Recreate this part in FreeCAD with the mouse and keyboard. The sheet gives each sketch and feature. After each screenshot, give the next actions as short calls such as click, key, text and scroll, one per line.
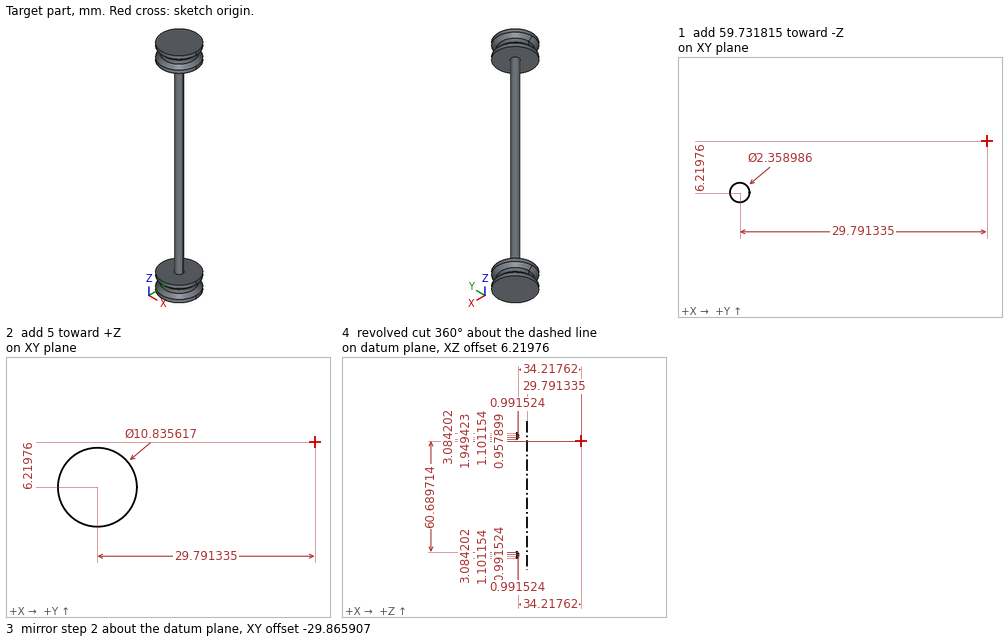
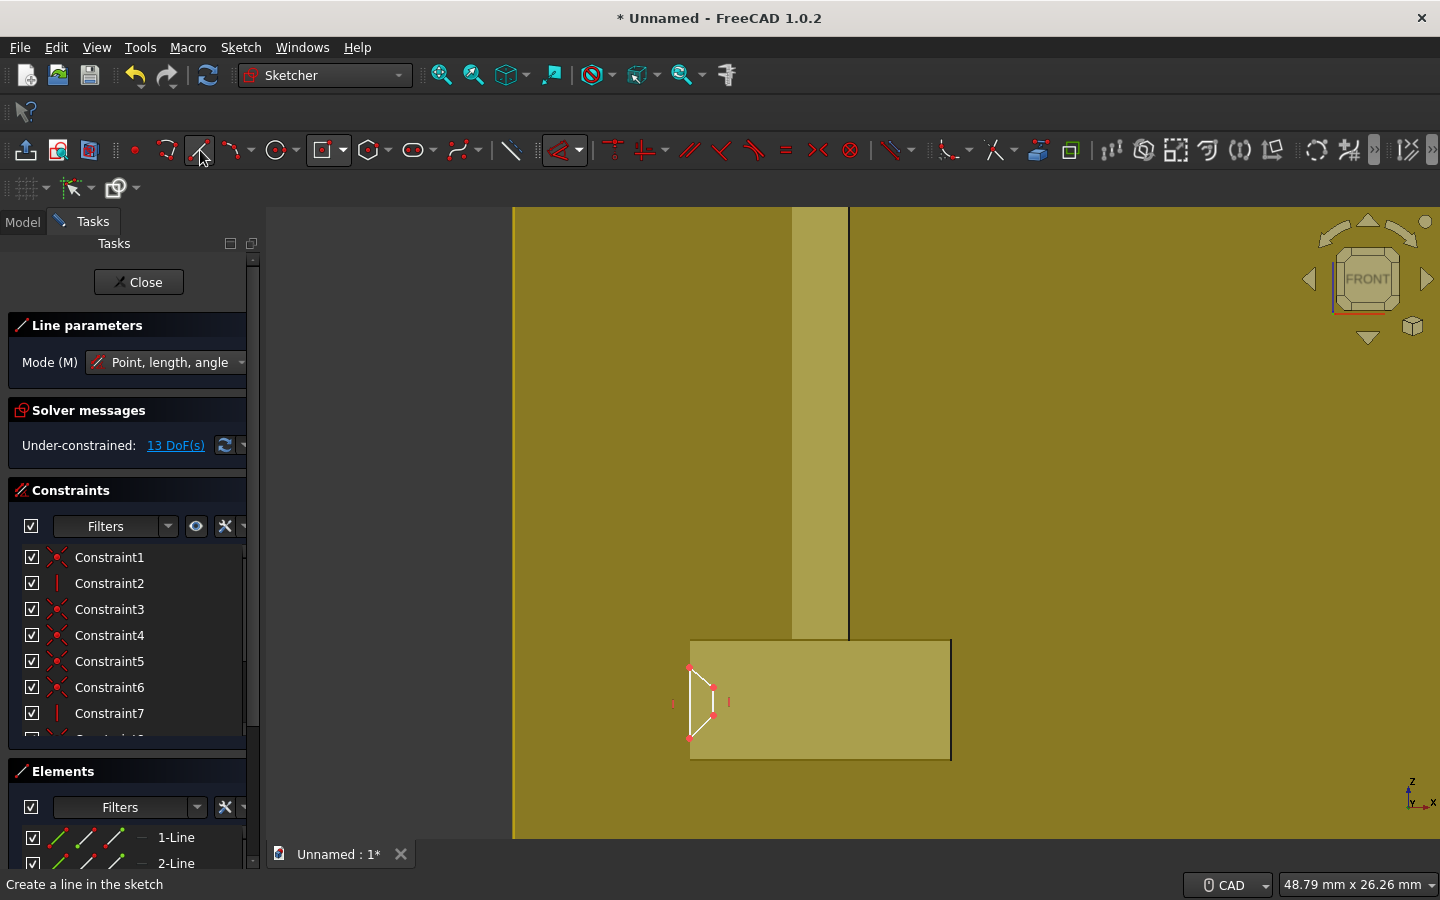
scroll(701, 675, down, 8)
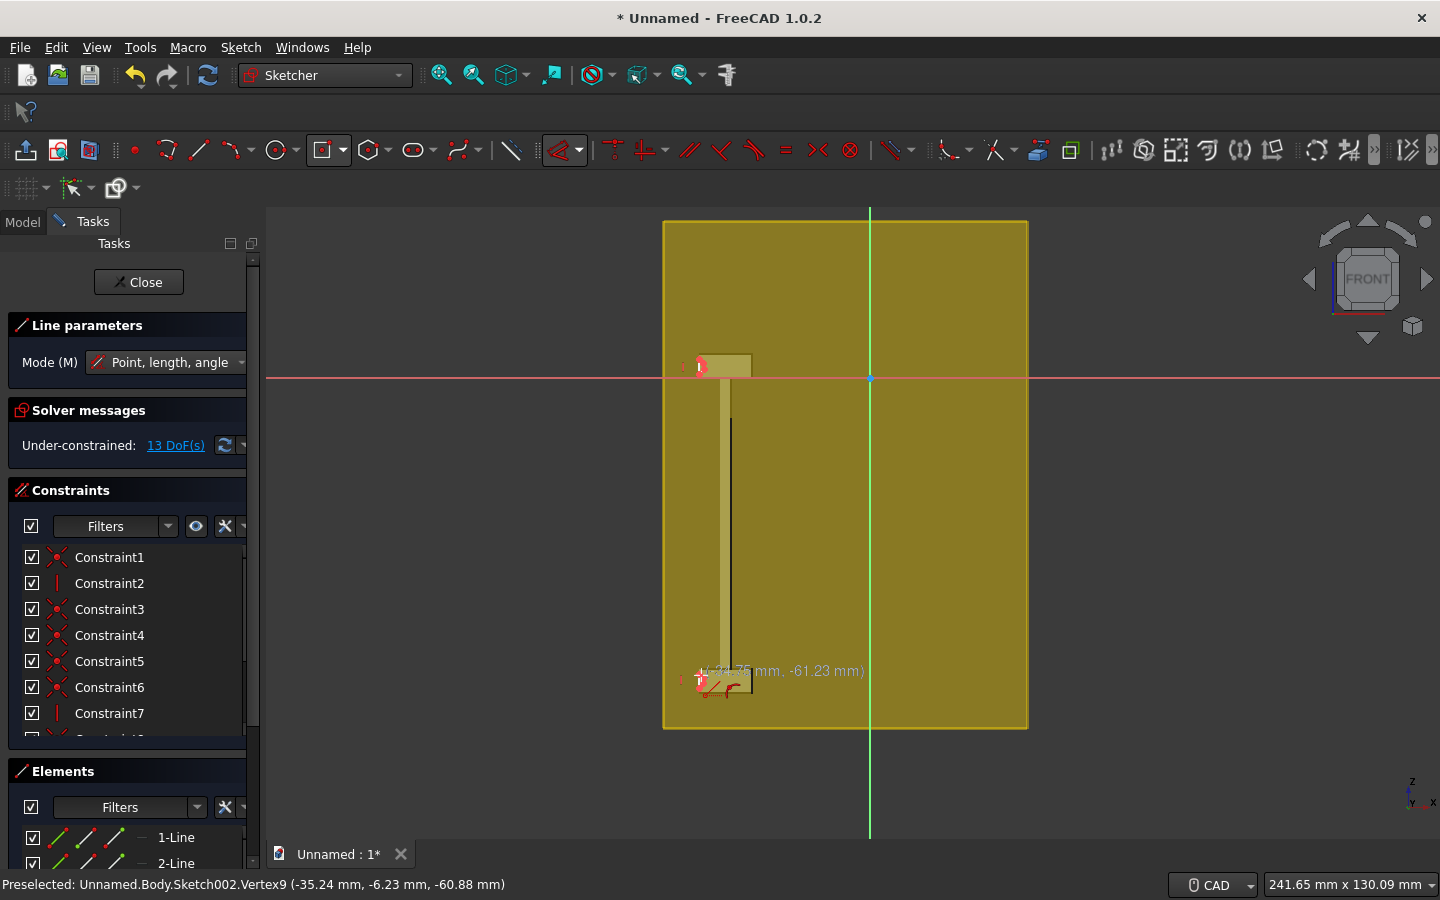
click(725, 326)
click(725, 721)
key(Escape)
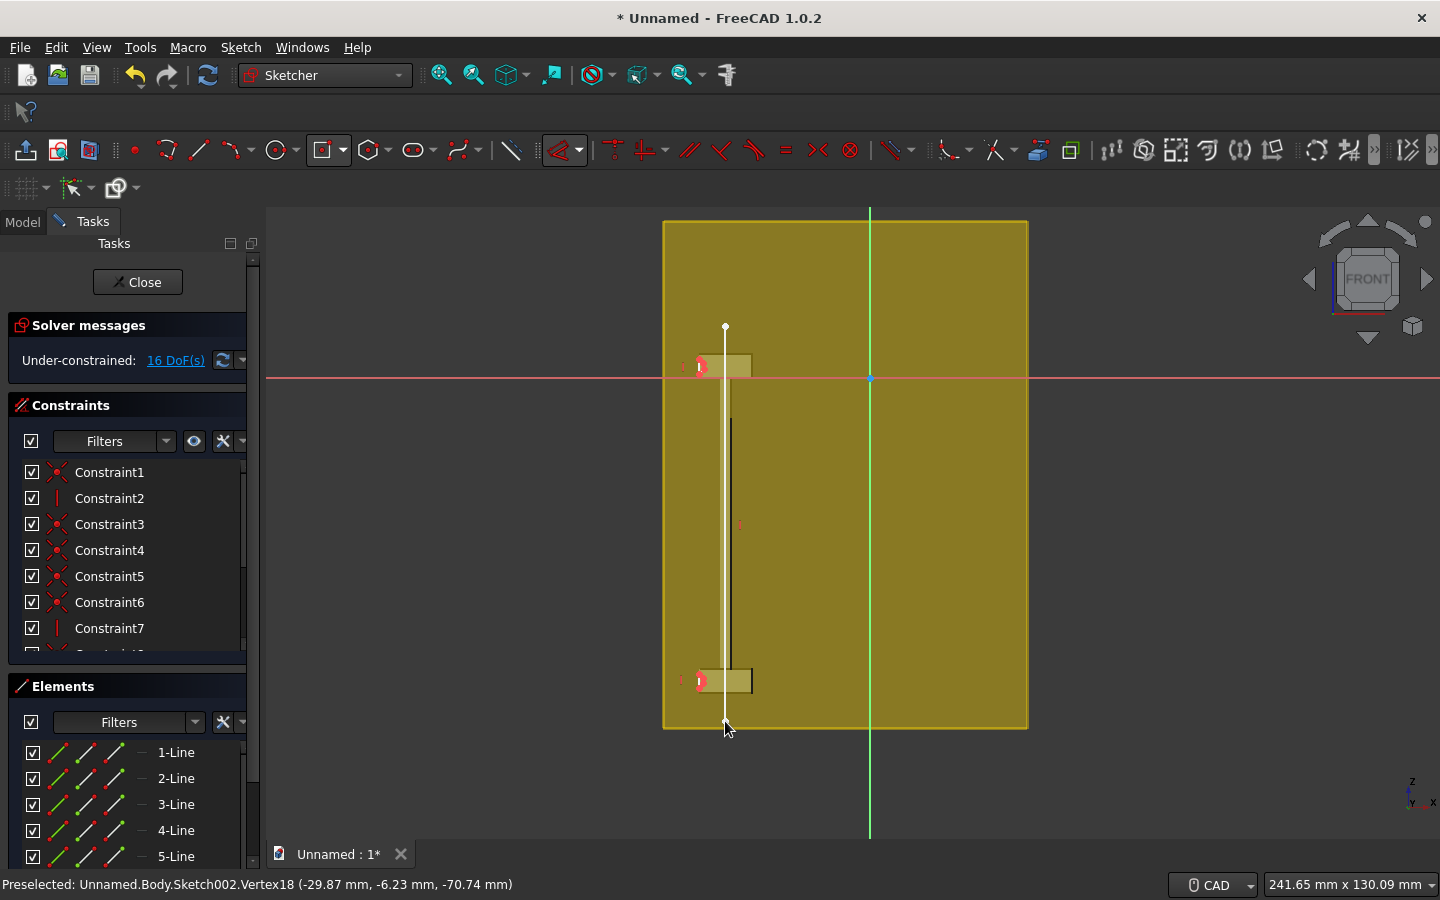
click(725, 445)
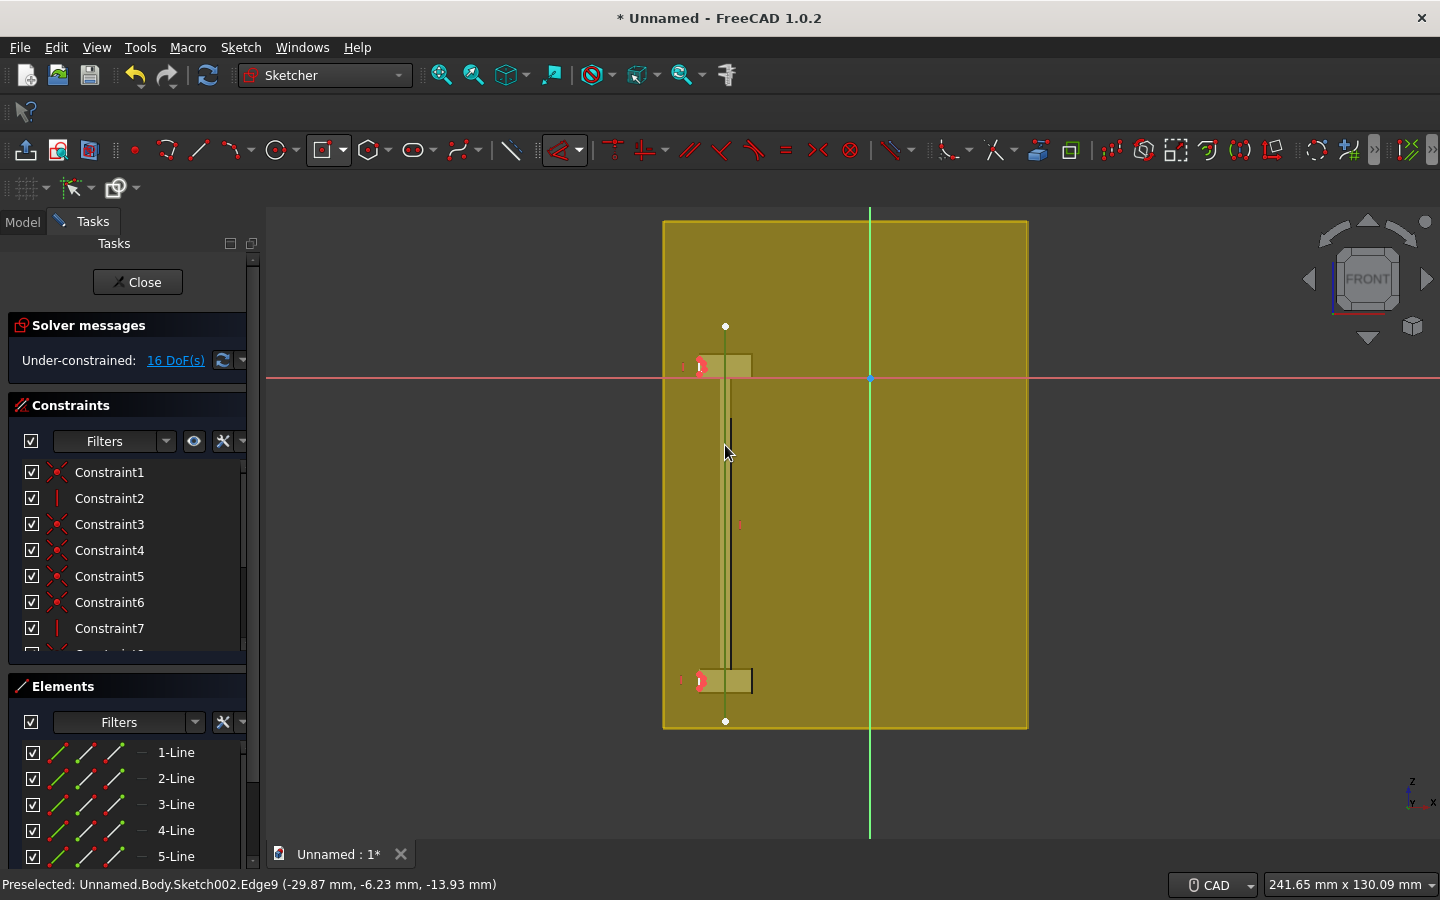
click(512, 150)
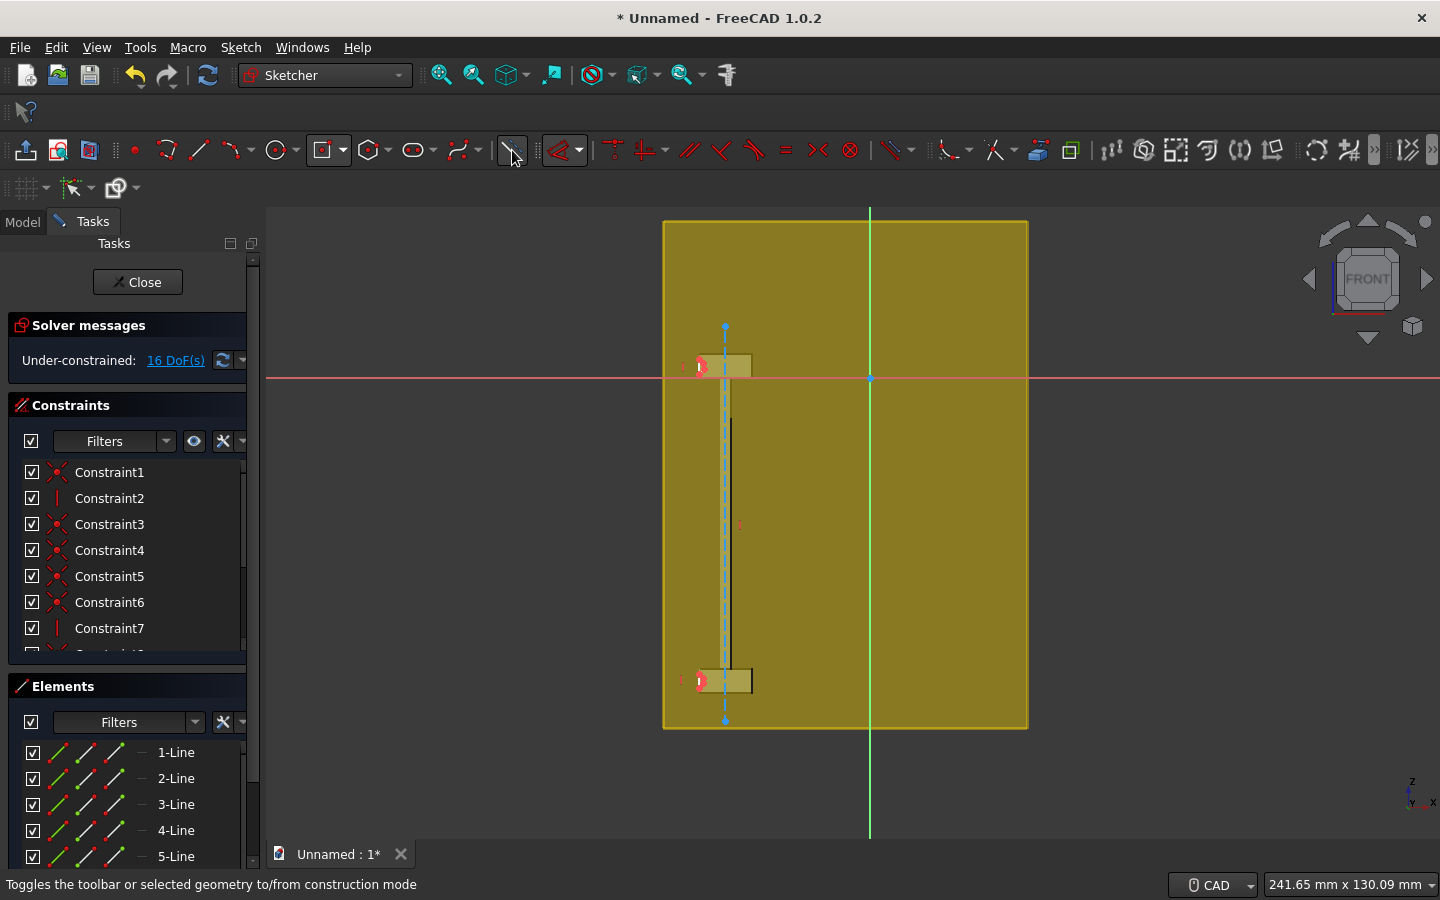
scroll(704, 367, up, 9)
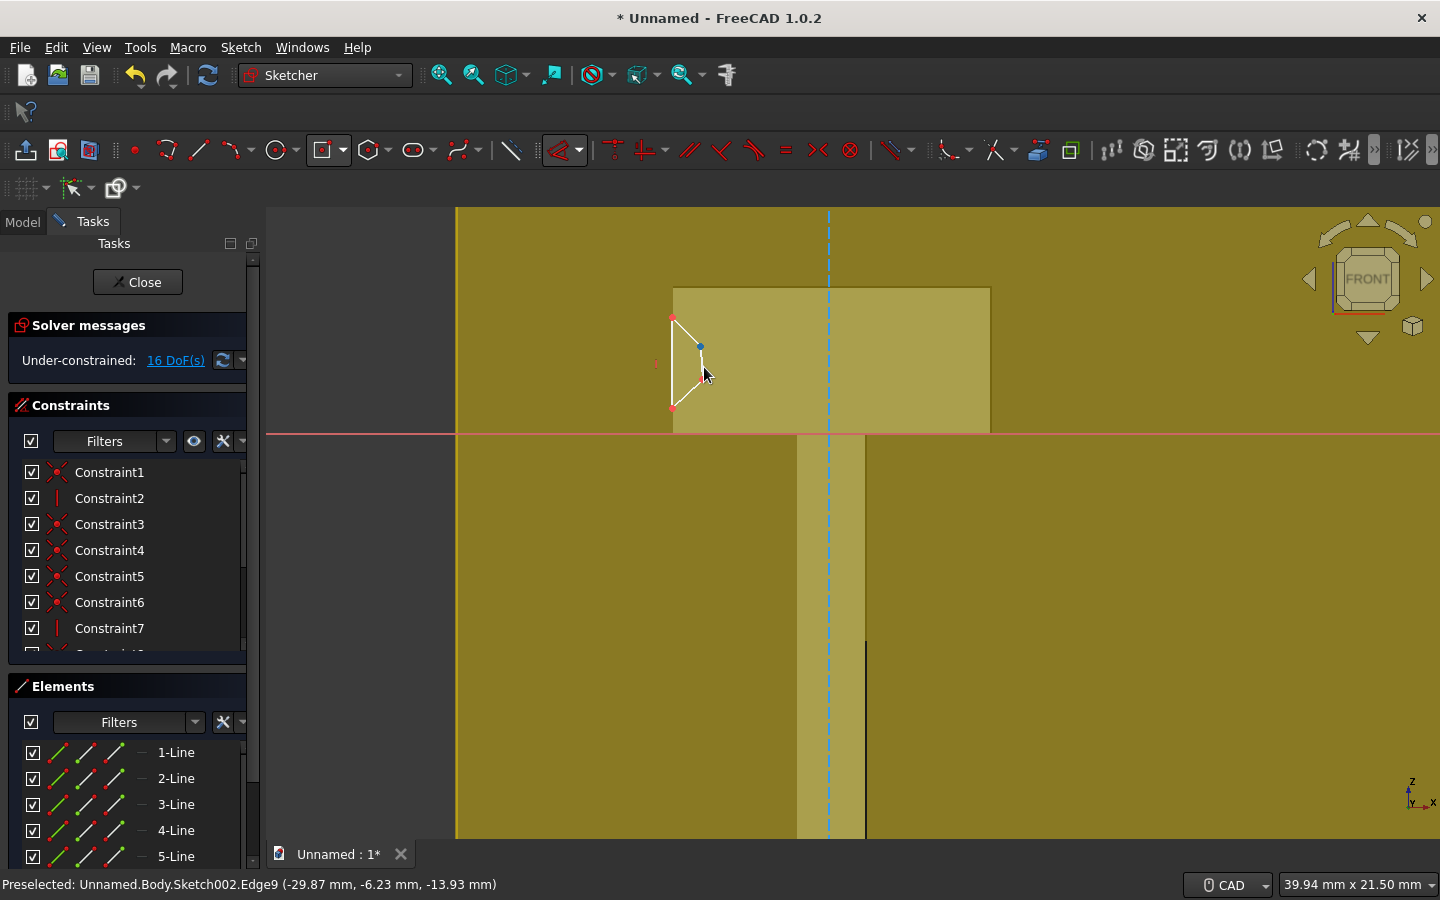
click(702, 363)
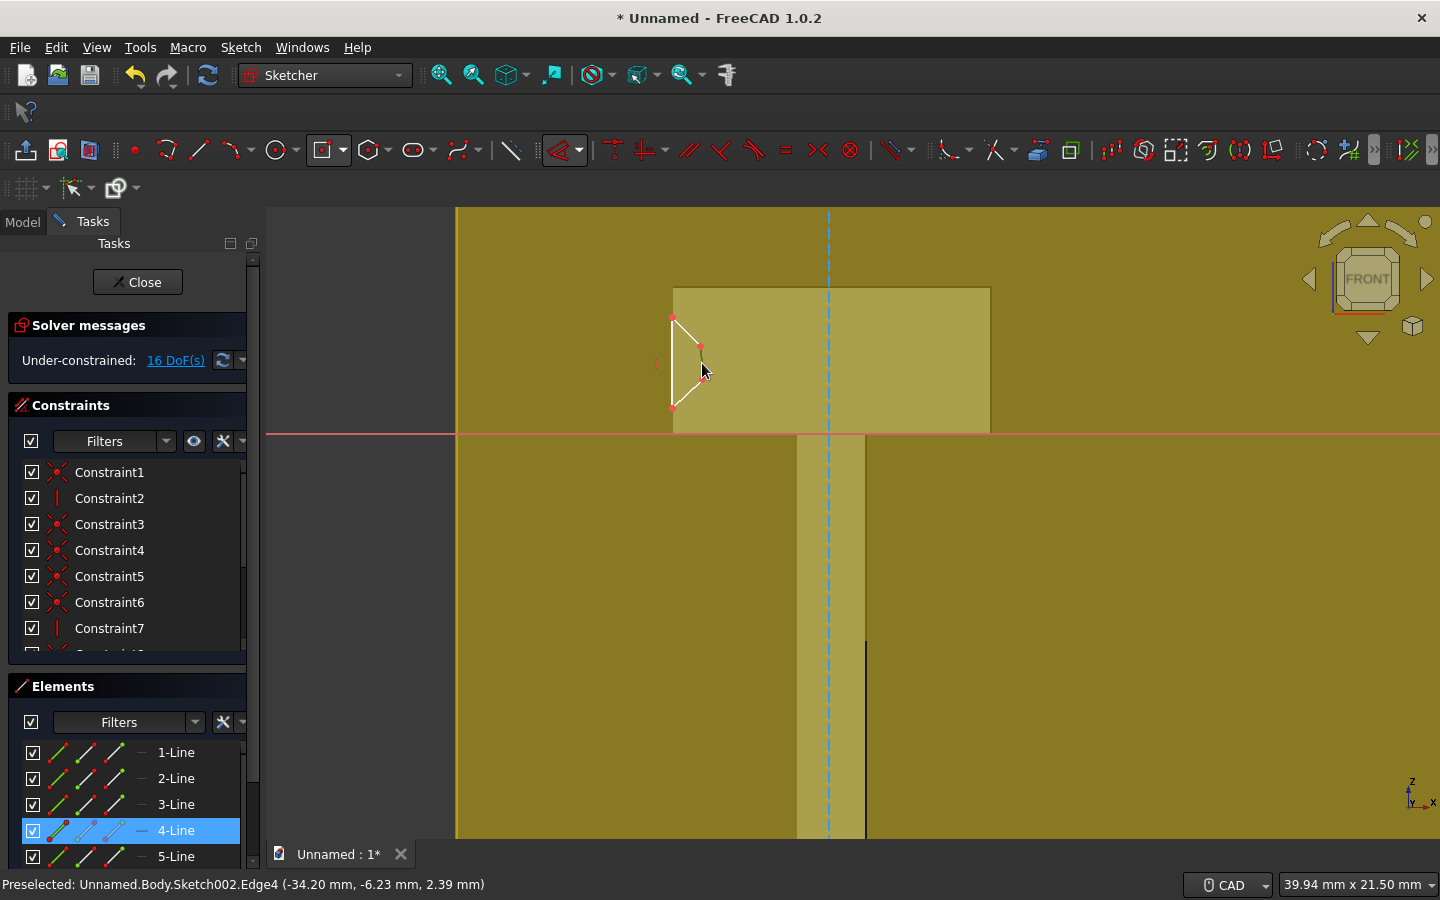
click(668, 150)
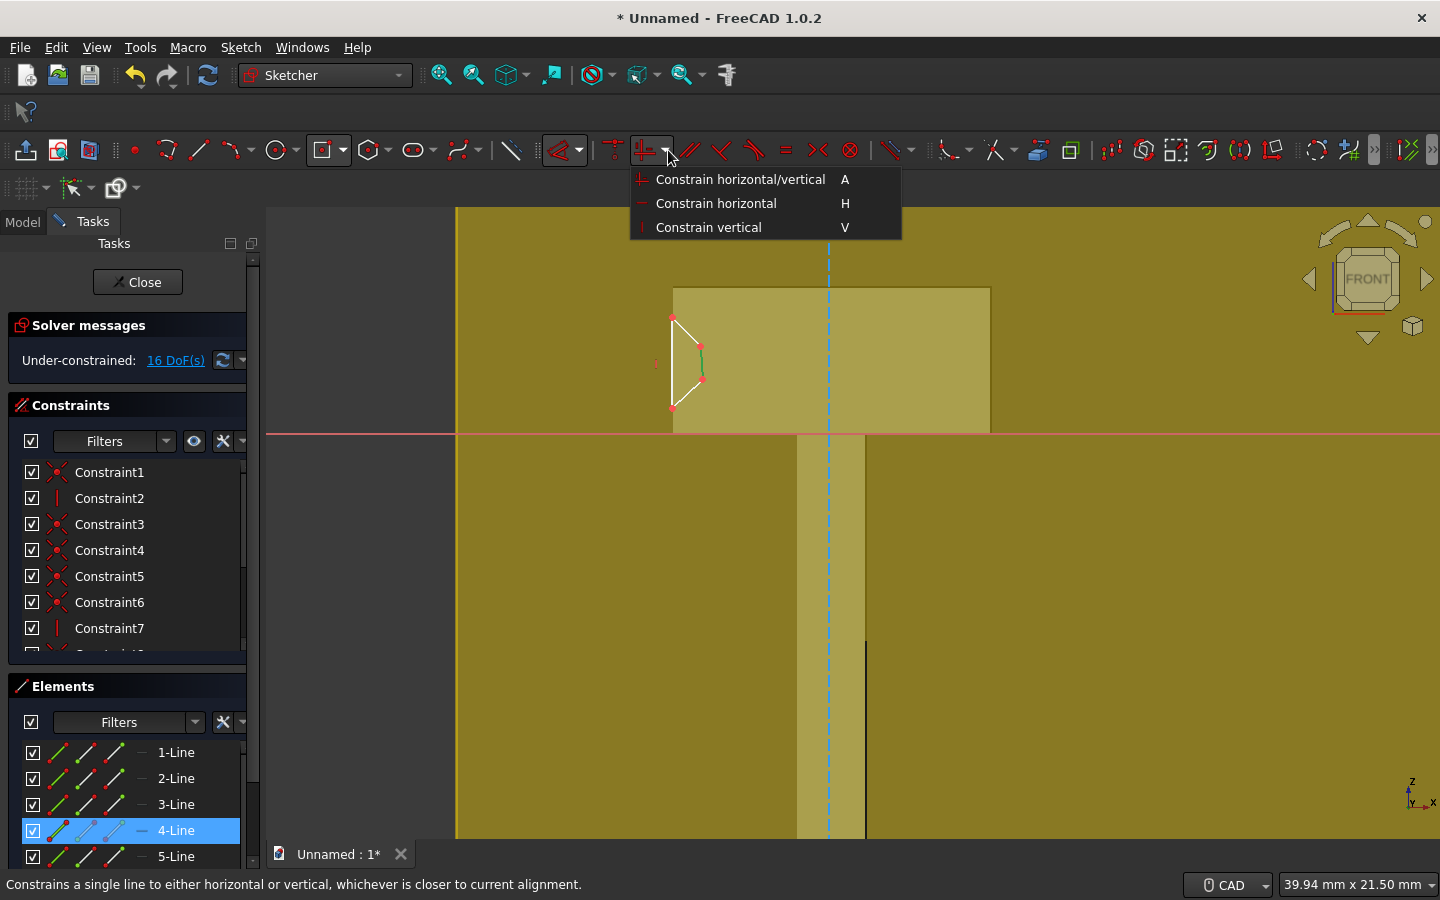
click(766, 227)